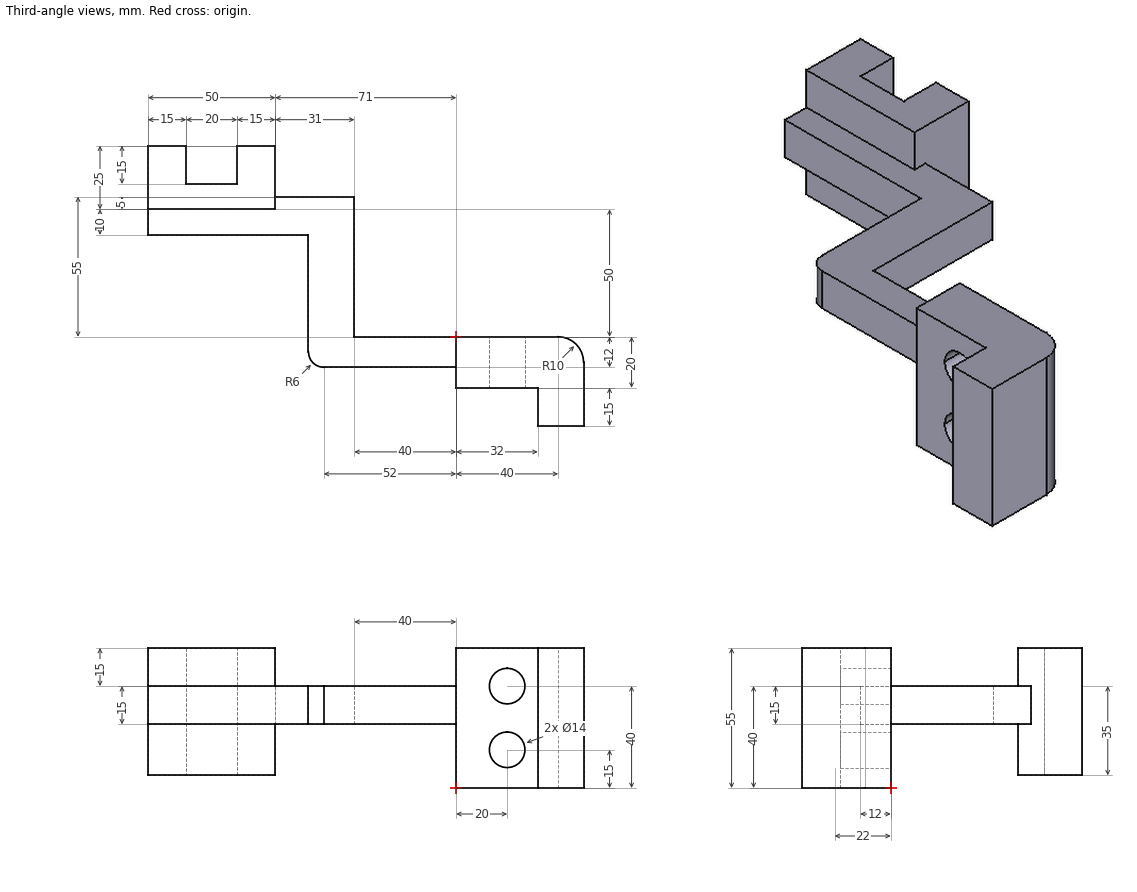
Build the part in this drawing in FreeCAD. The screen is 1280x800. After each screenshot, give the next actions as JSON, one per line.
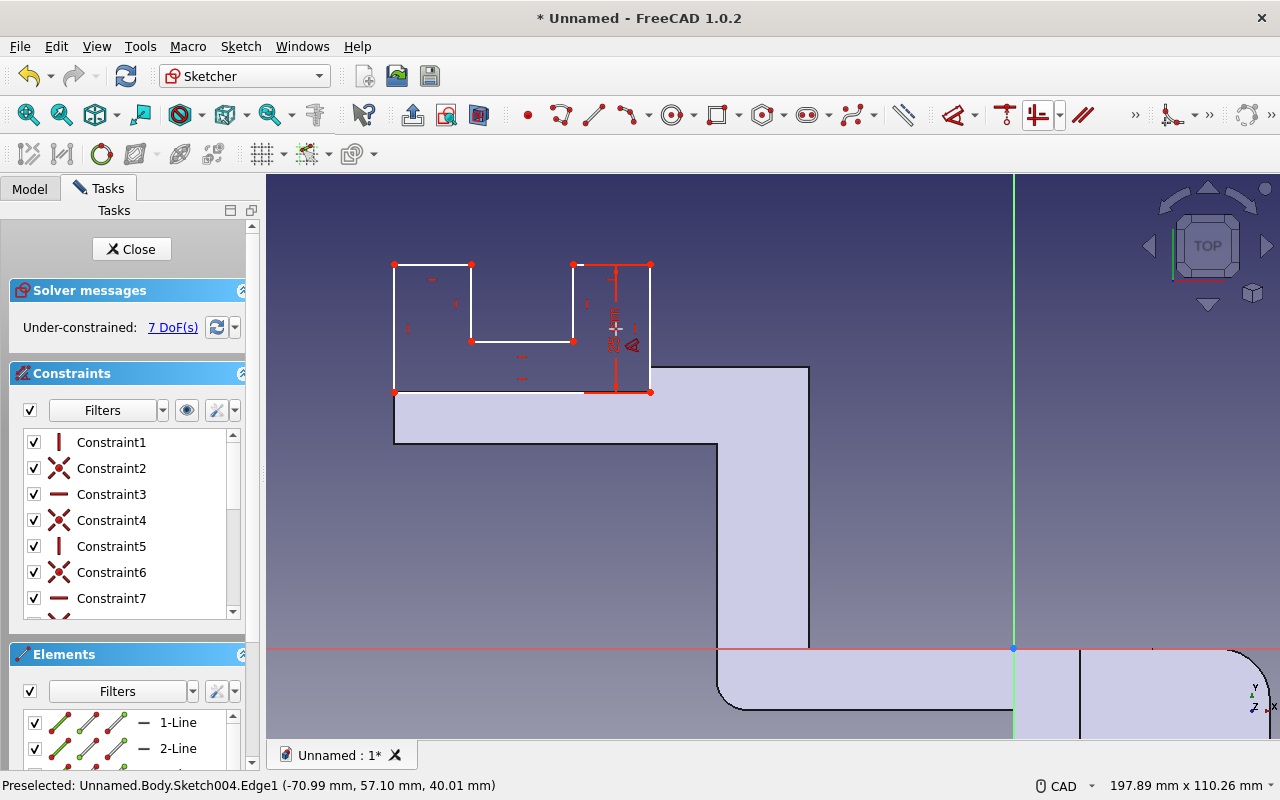
{"action": "left_click", "coordinate": [627, 265]}
{"action": "left_click", "coordinate": [611, 231]}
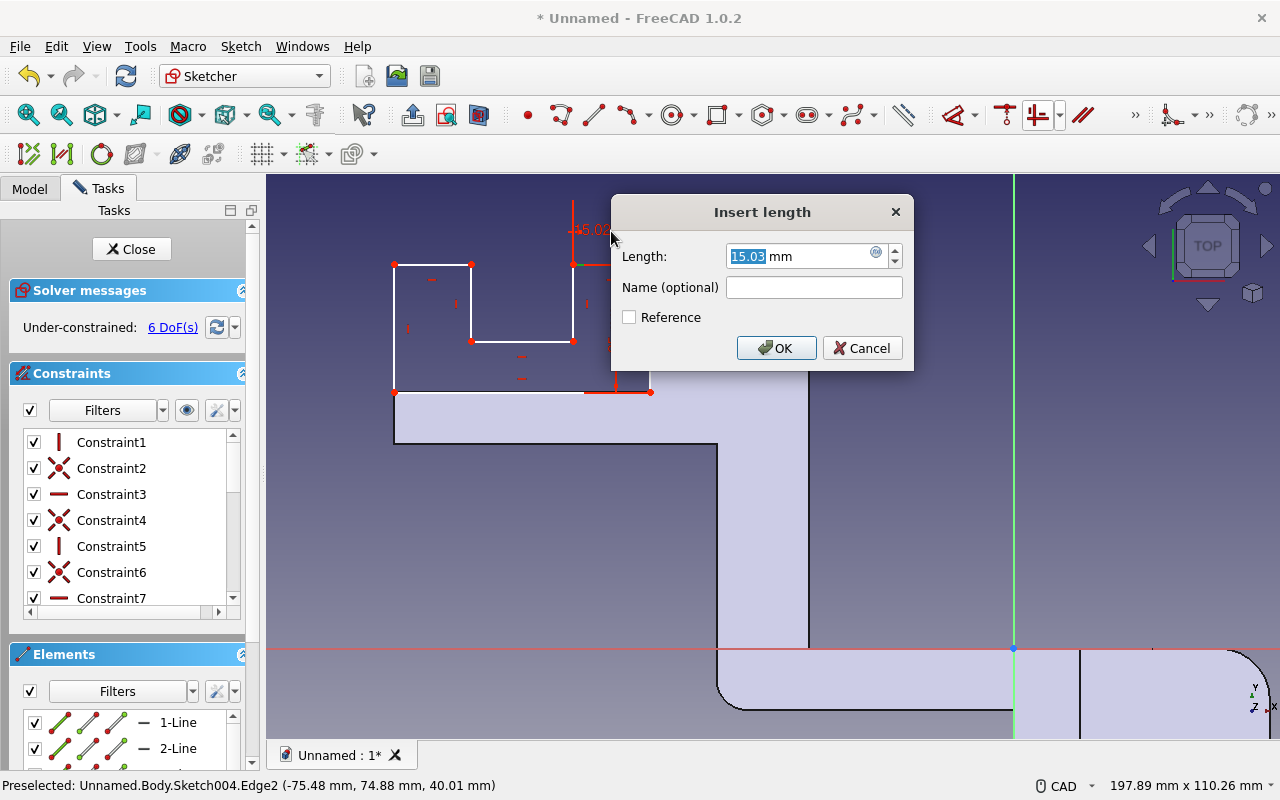
{"action": "type", "text": "15"}
{"action": "key", "text": "Return"}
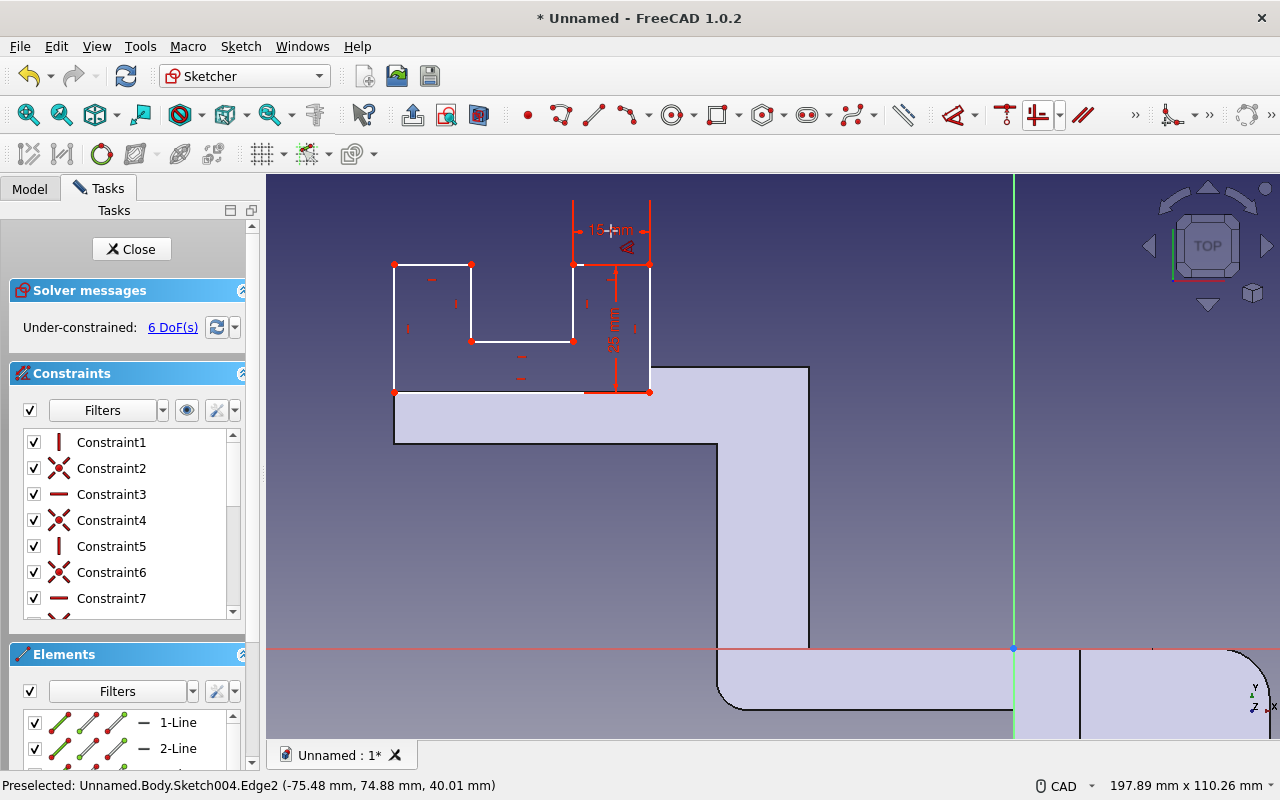
{"action": "left_click", "coordinate": [573, 288]}
{"action": "left_click", "coordinate": [539, 303]}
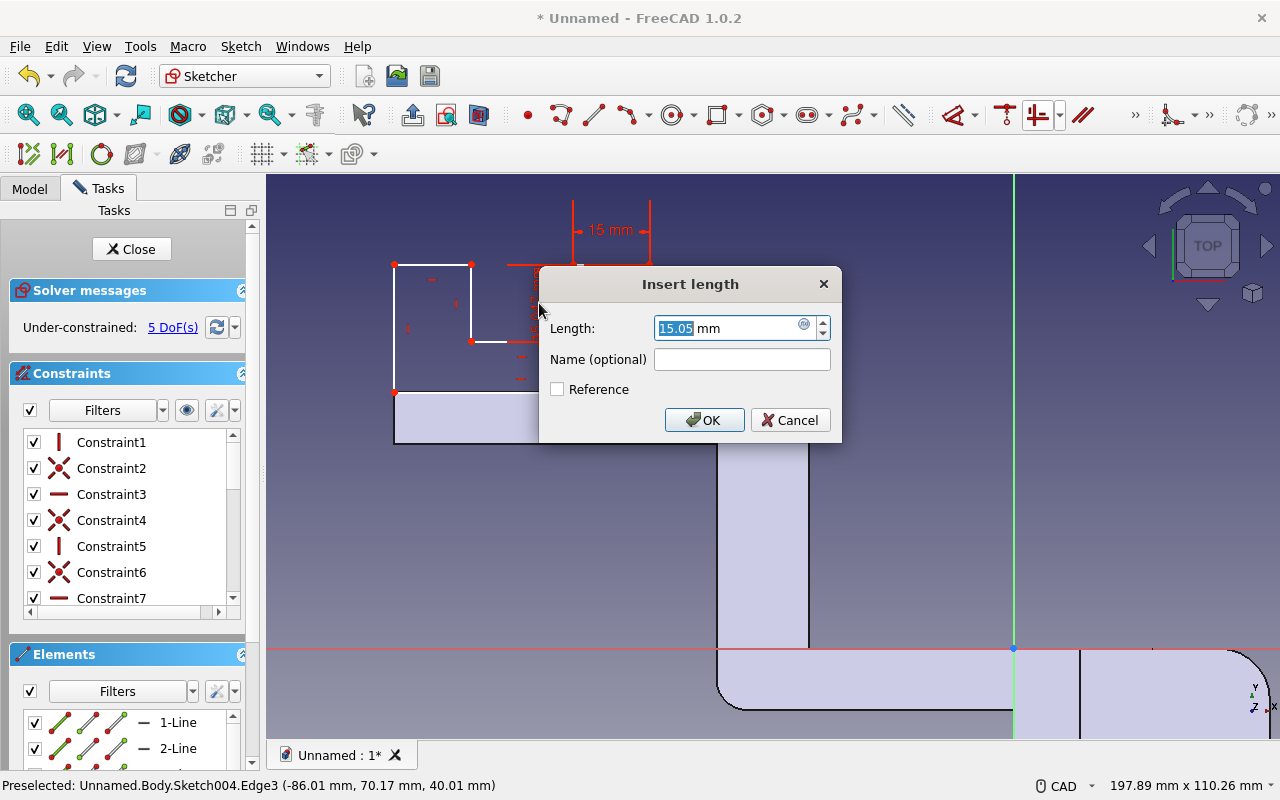
{"action": "type", "text": "15"}
{"action": "key", "text": "Return"}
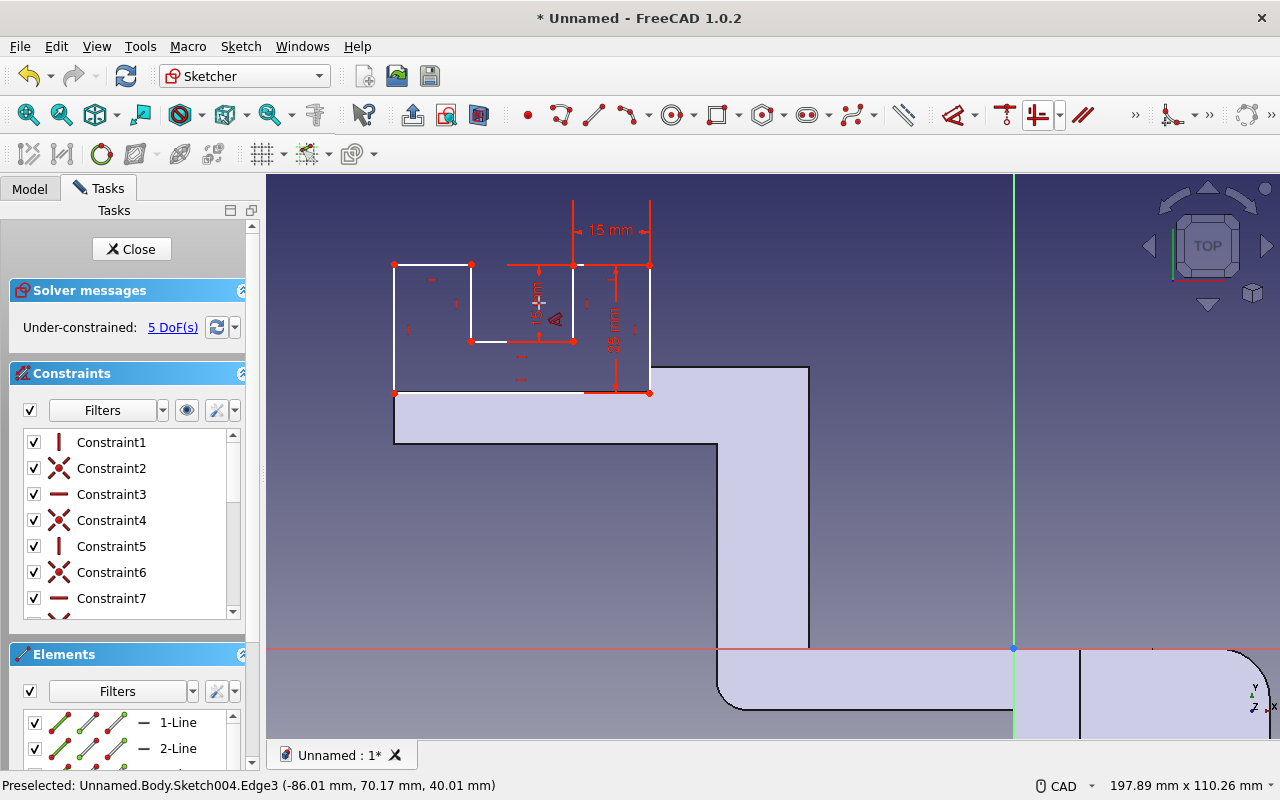
{"action": "left_click", "coordinate": [542, 342]}
{"action": "left_click", "coordinate": [522, 376]}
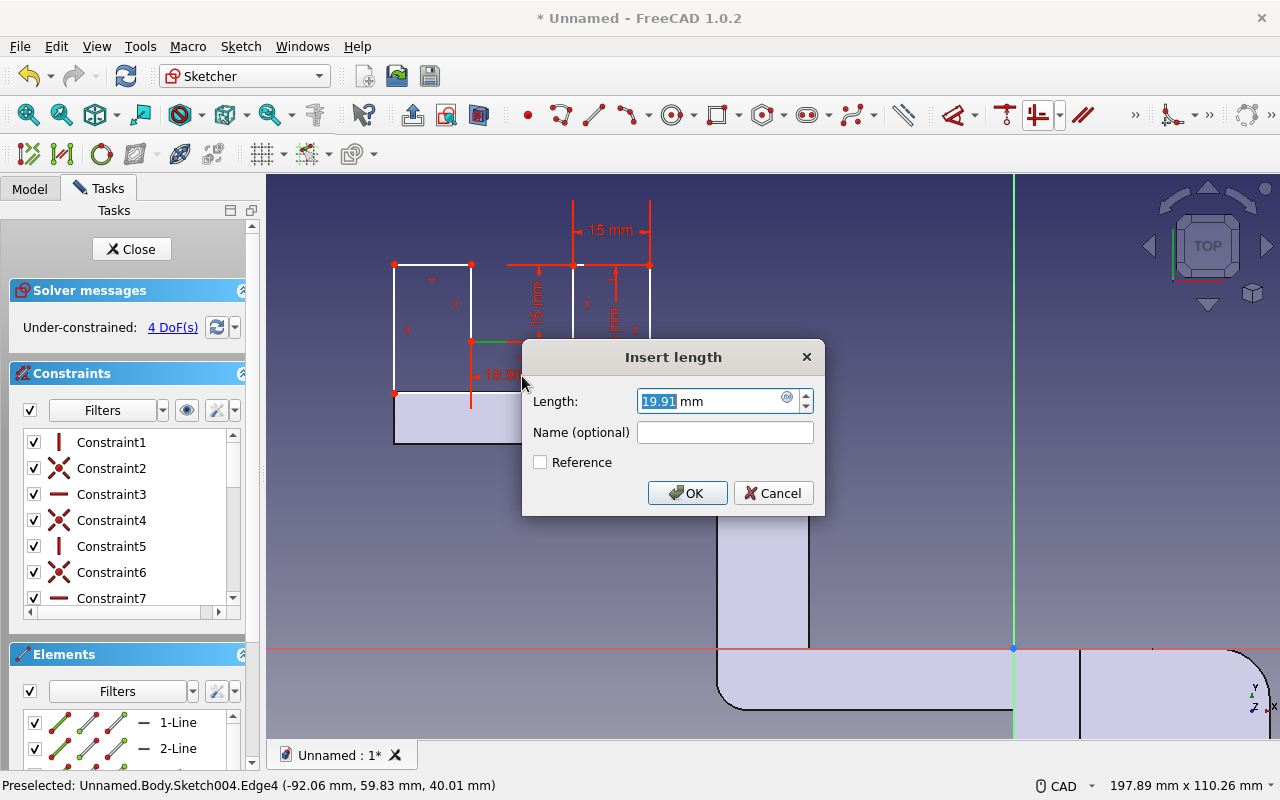
{"action": "type", "text": "20"}
{"action": "key", "text": "Return"}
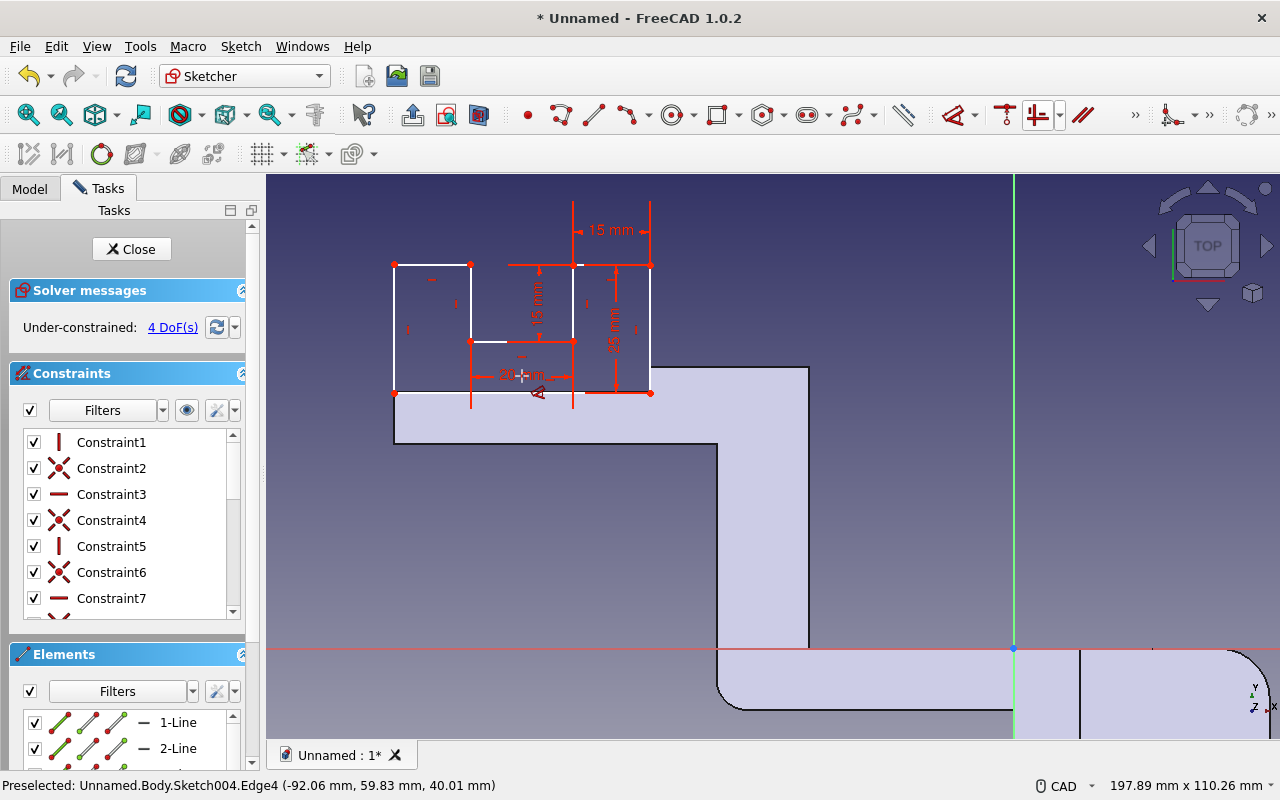
{"action": "left_click", "coordinate": [471, 319]}
{"action": "left_click", "coordinate": [437, 304]}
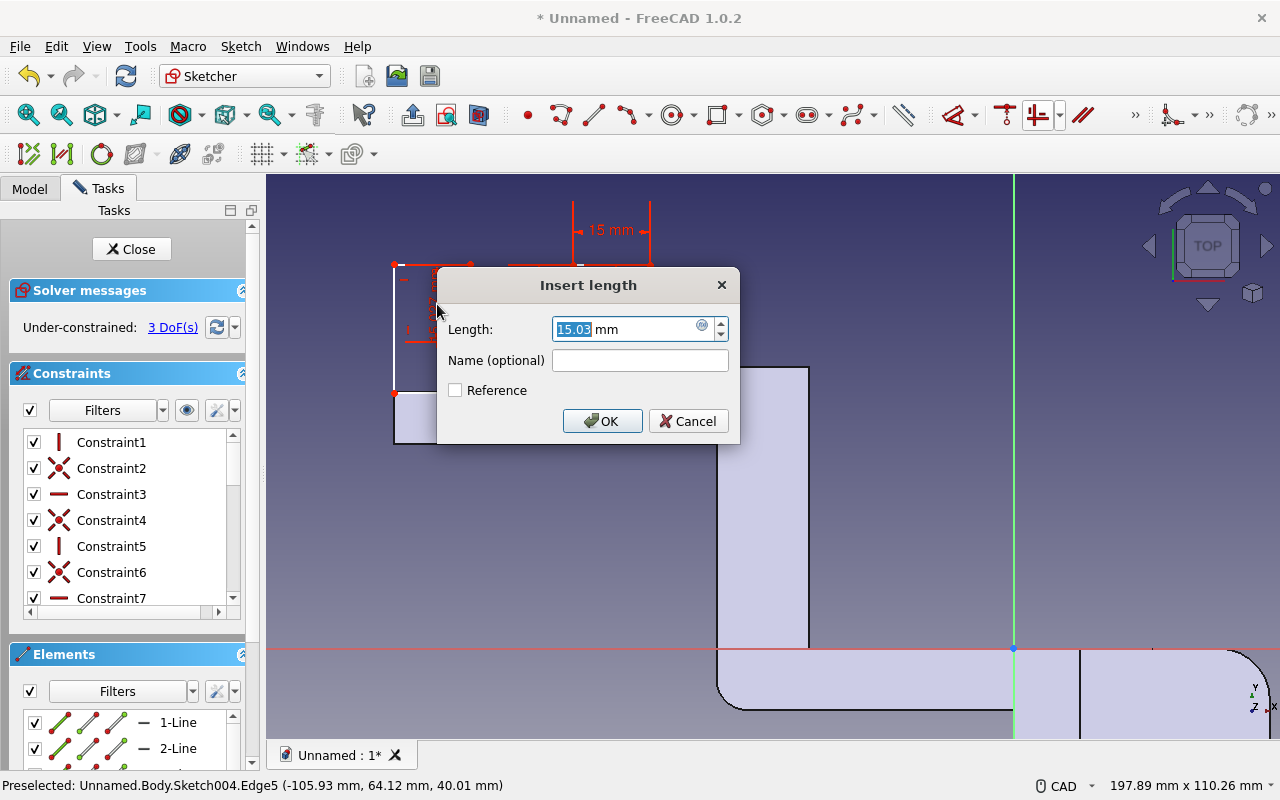
{"action": "type", "text": "15"}
{"action": "key", "text": "Return"}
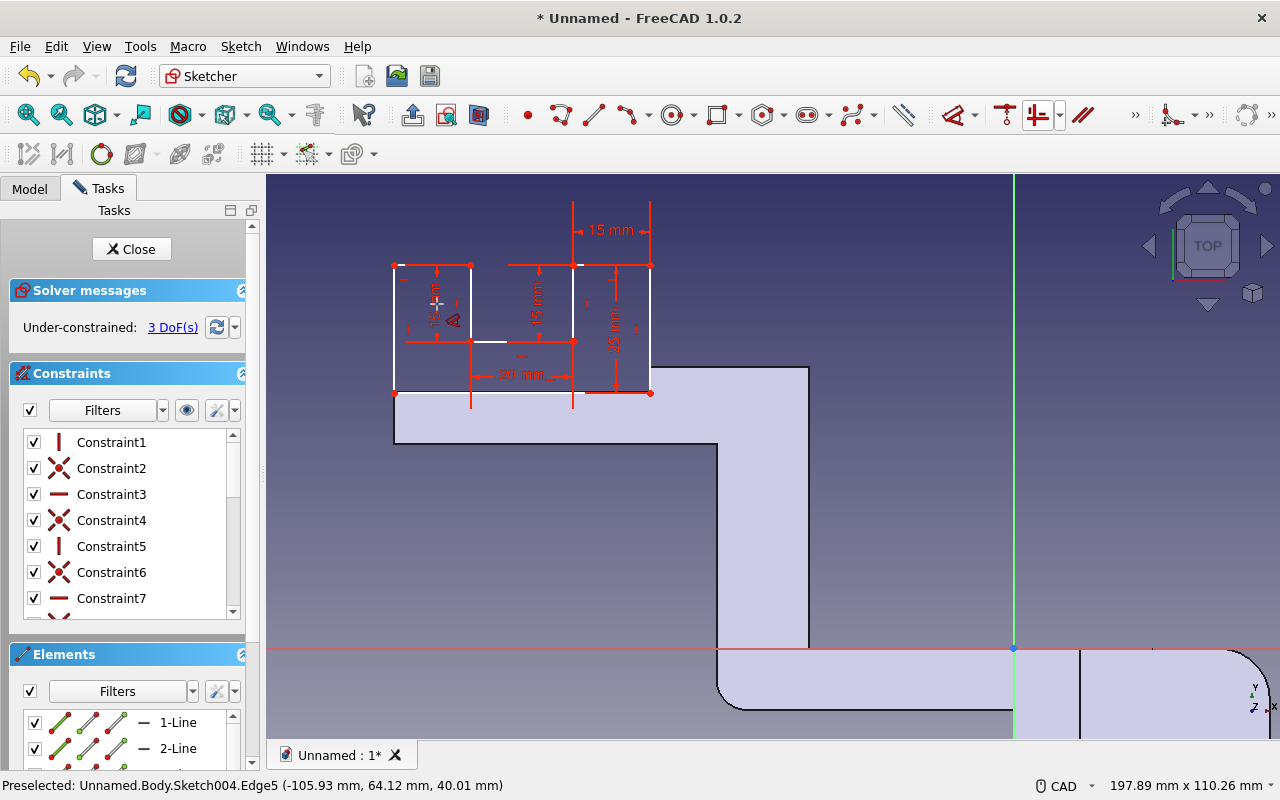
{"action": "left_click", "coordinate": [448, 265]}
{"action": "left_click", "coordinate": [432, 231]}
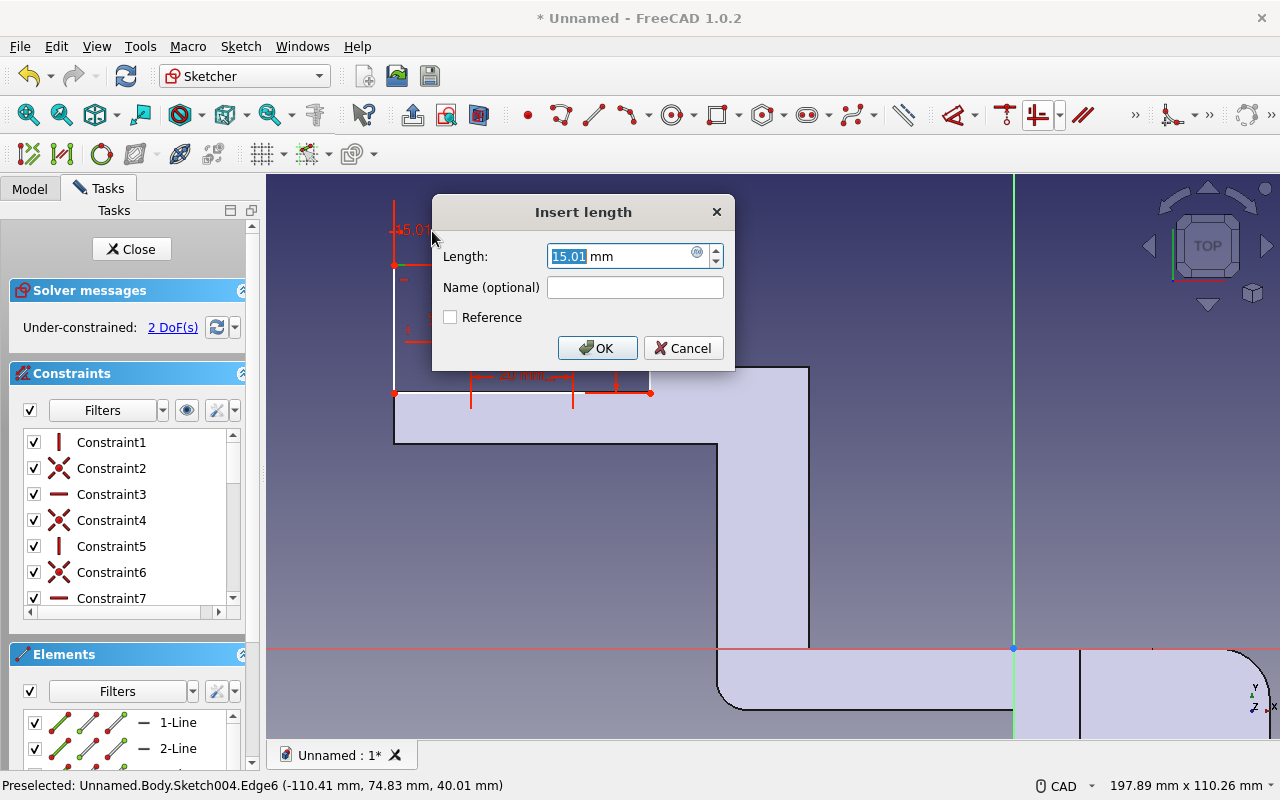
{"action": "type", "text": "15"}
{"action": "key", "text": "Return"}